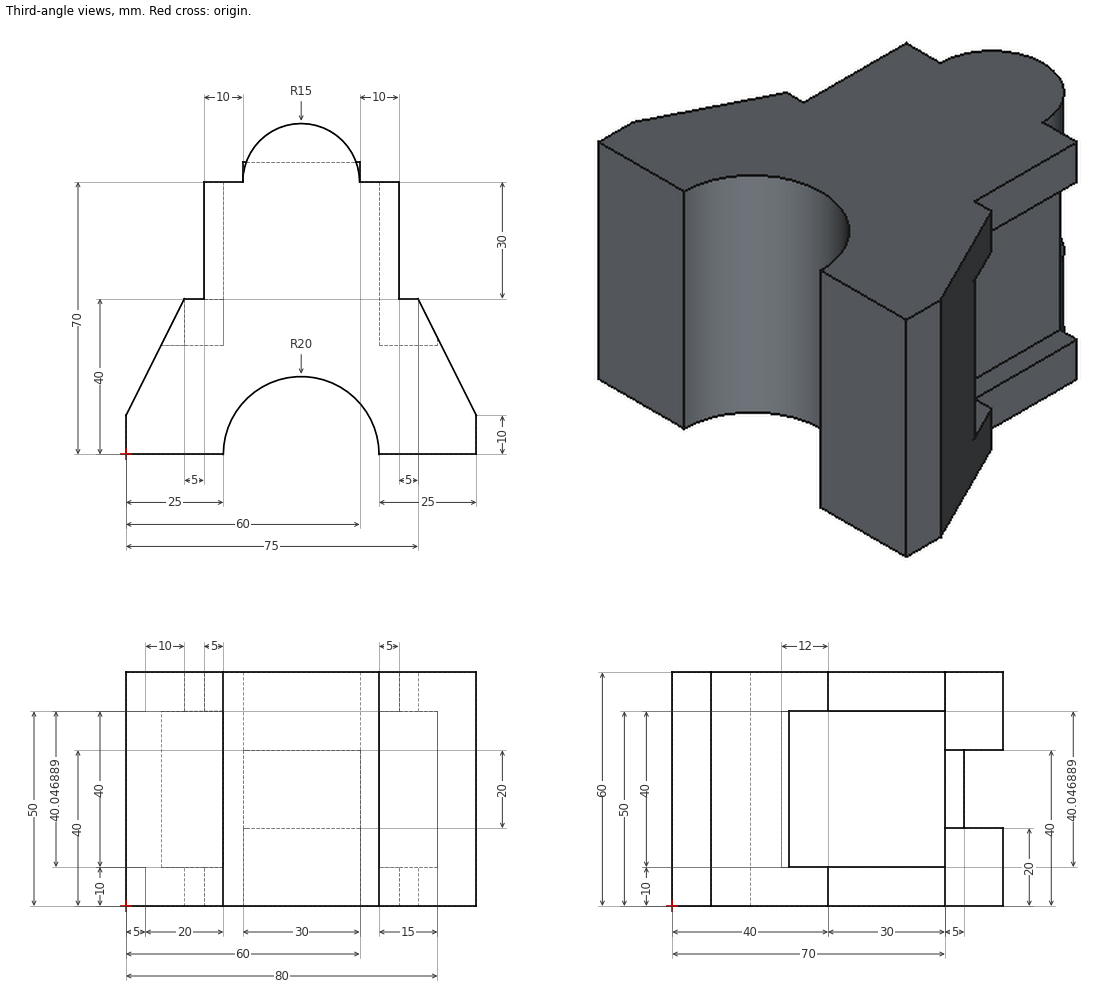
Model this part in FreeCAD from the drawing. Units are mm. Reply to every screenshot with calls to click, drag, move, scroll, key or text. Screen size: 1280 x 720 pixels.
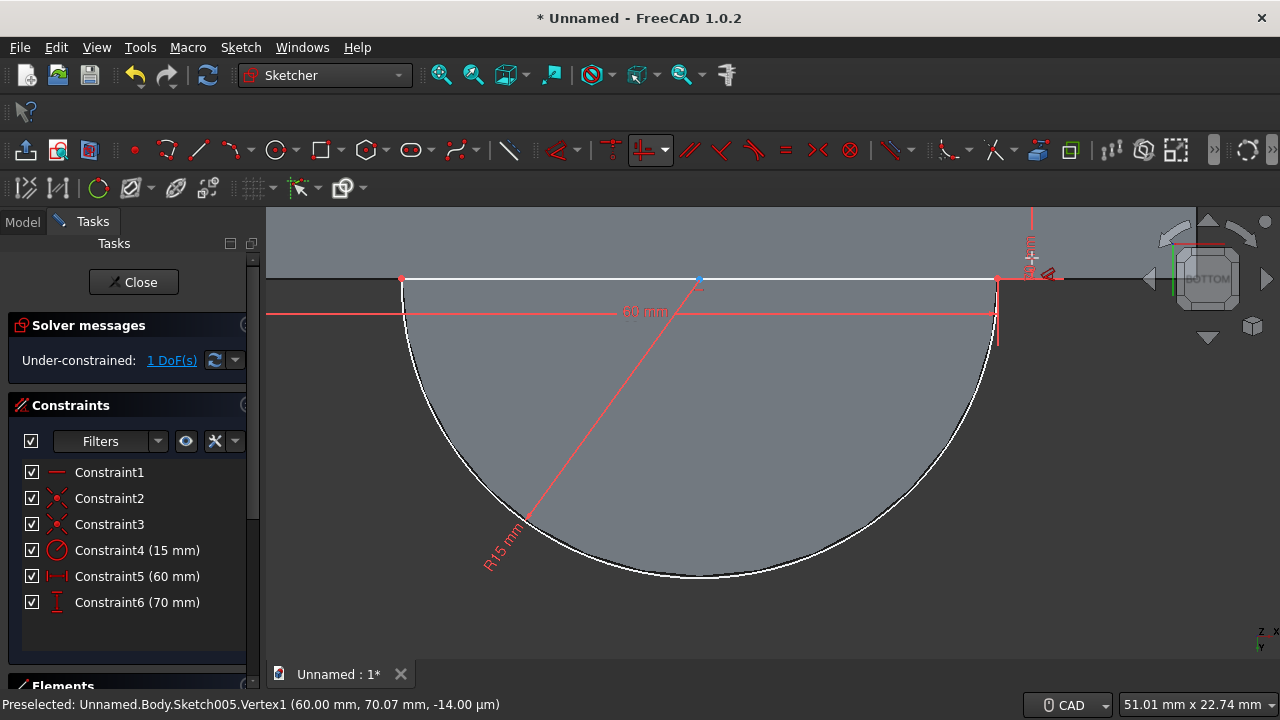
click(700, 280)
click(734, 257)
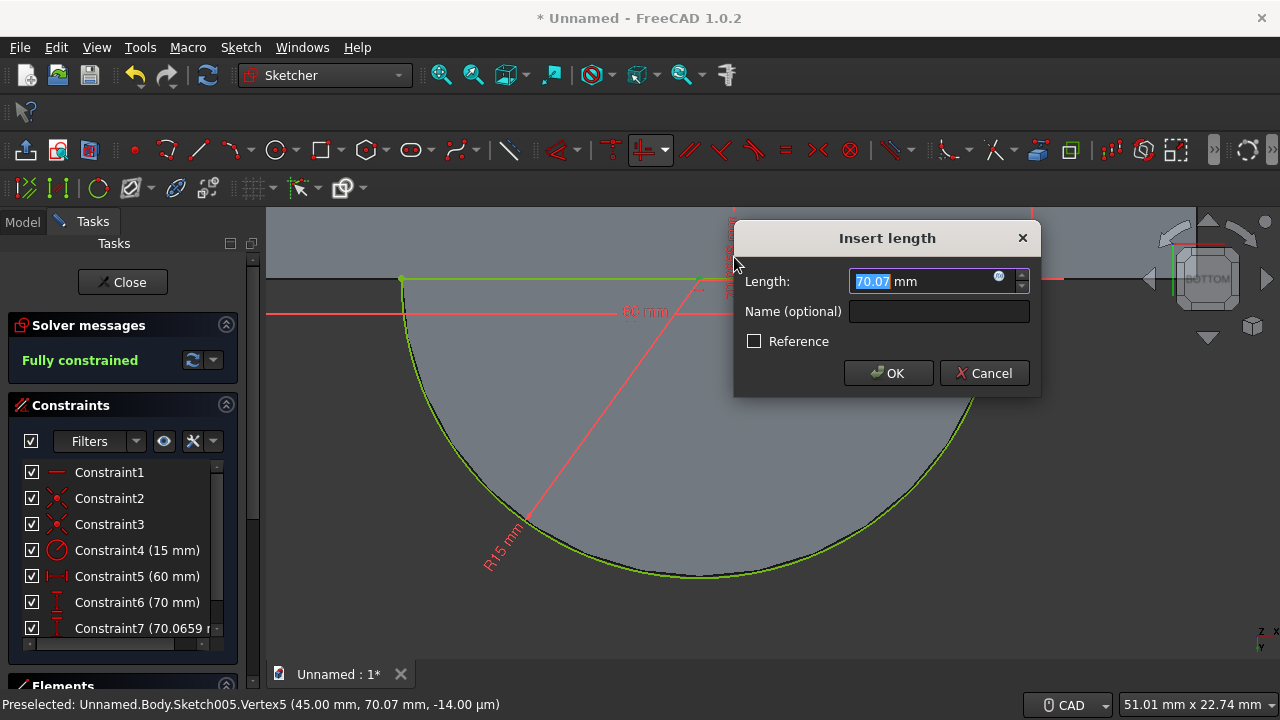
text(70)
key(Return)
key(Escape)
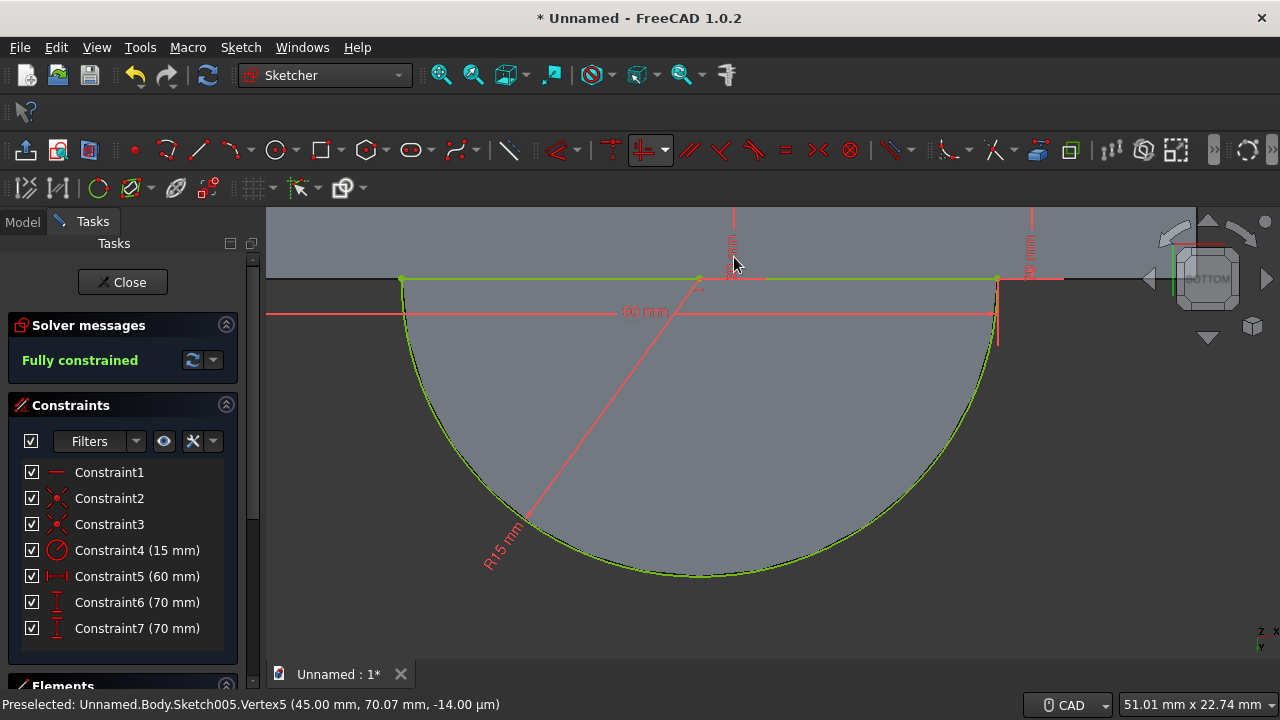
click(123, 282)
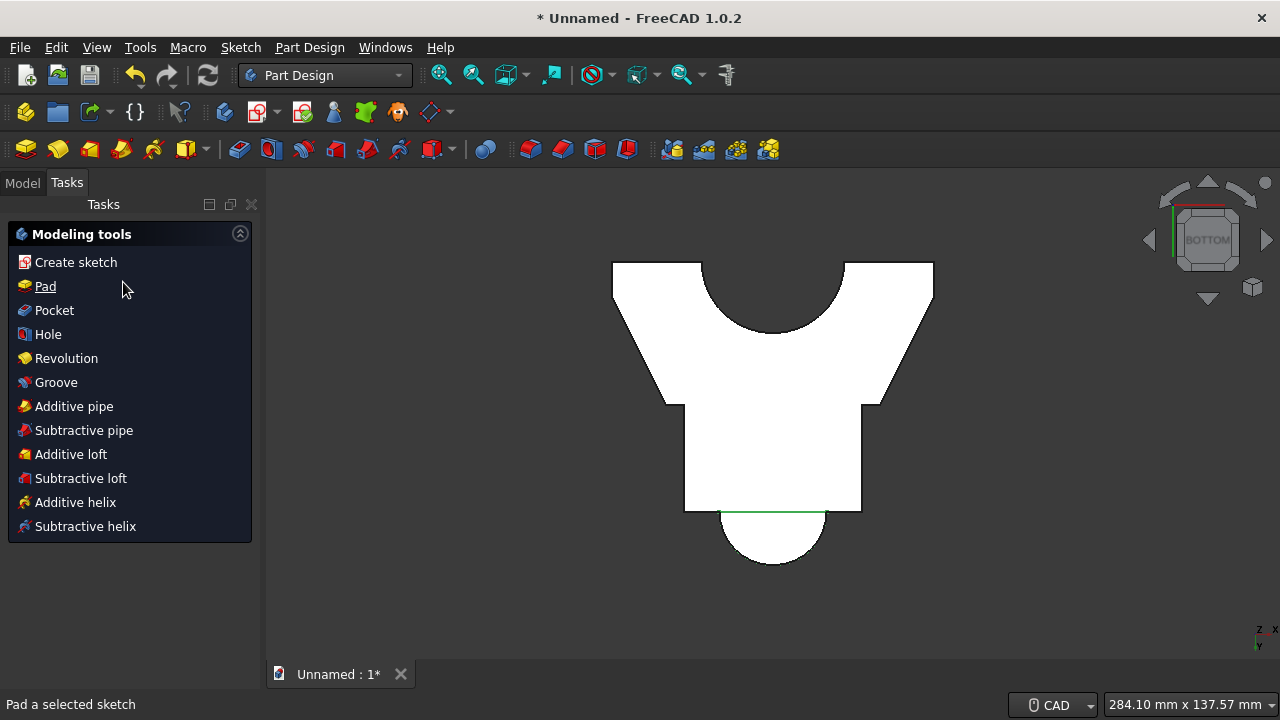
click(240, 150)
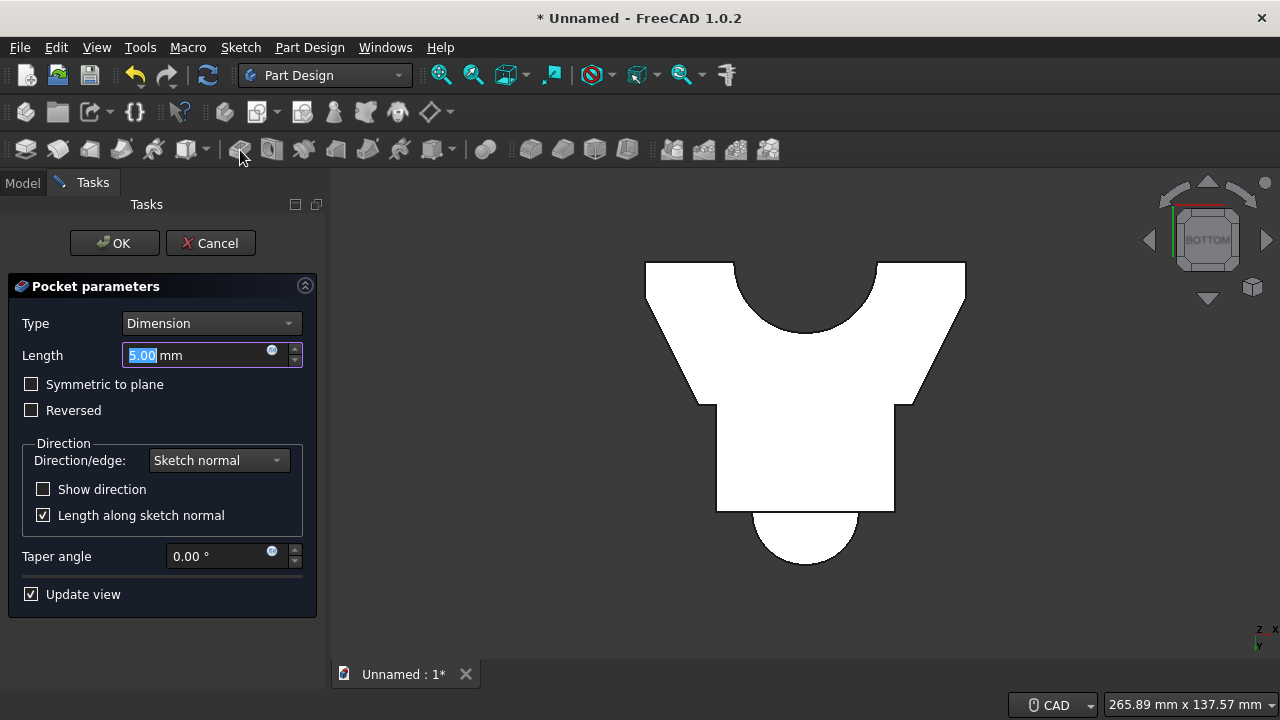
text(40)
key(Tab)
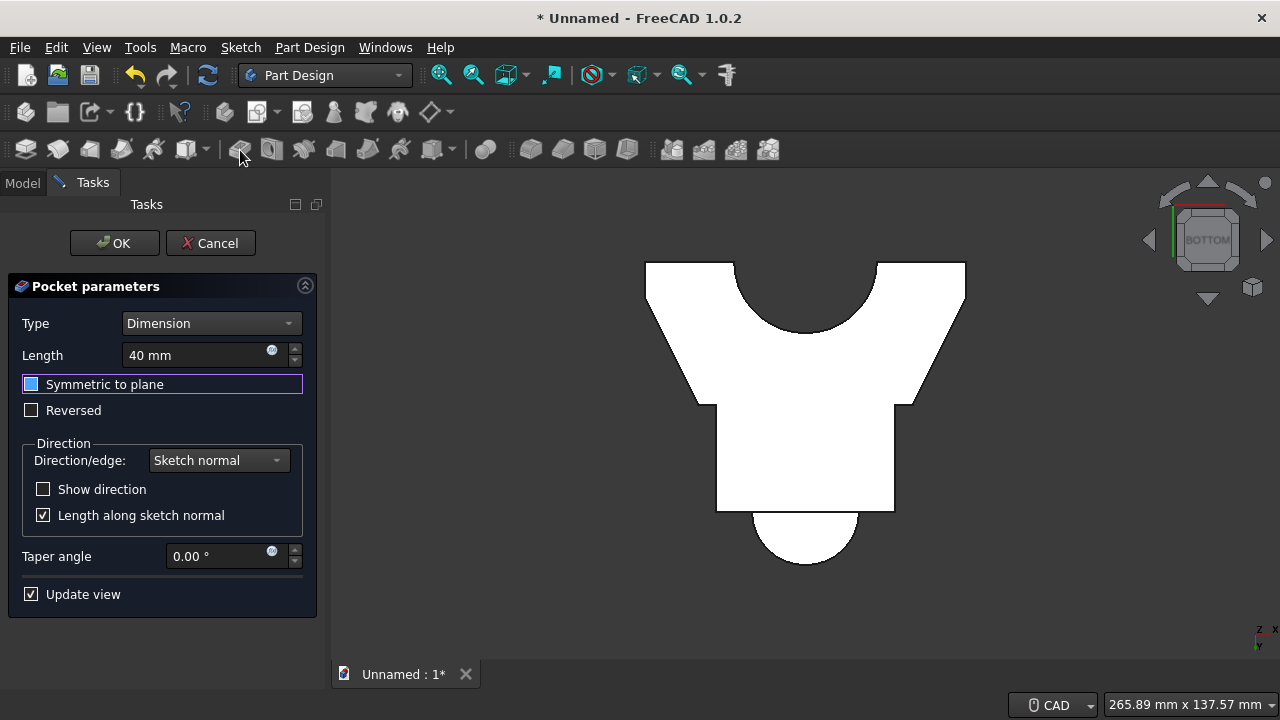
click(115, 243)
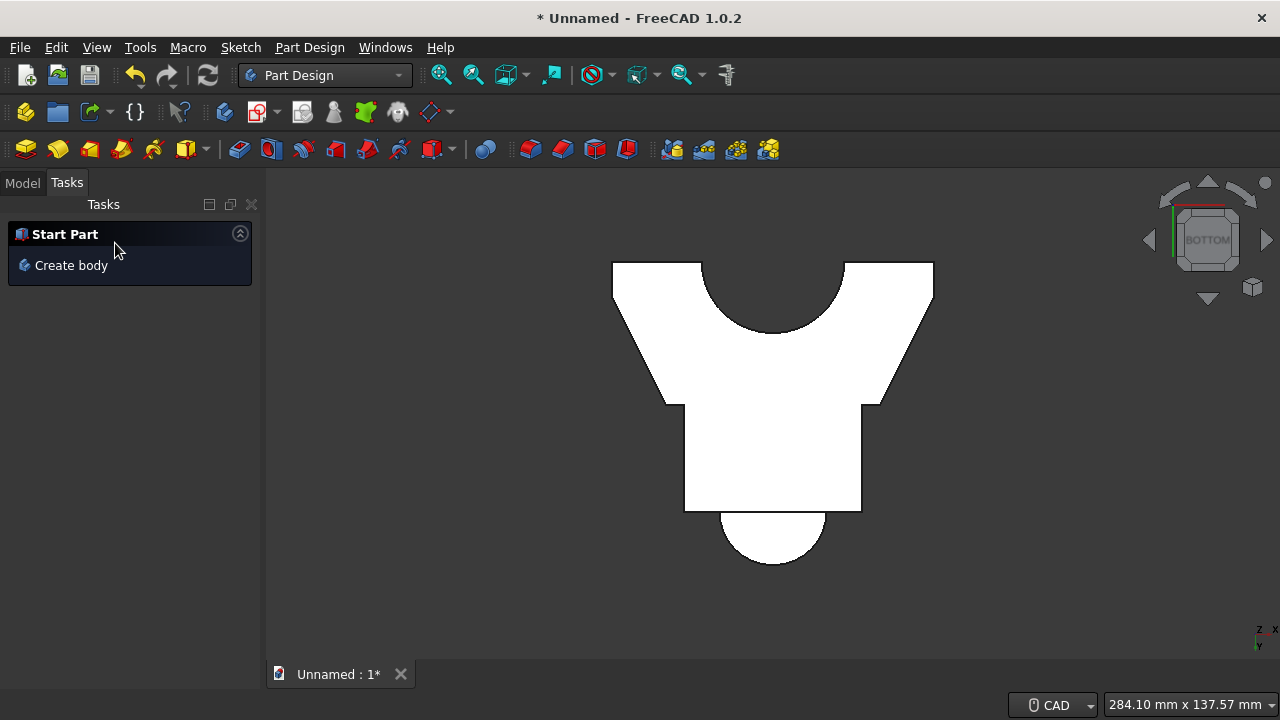
key(4)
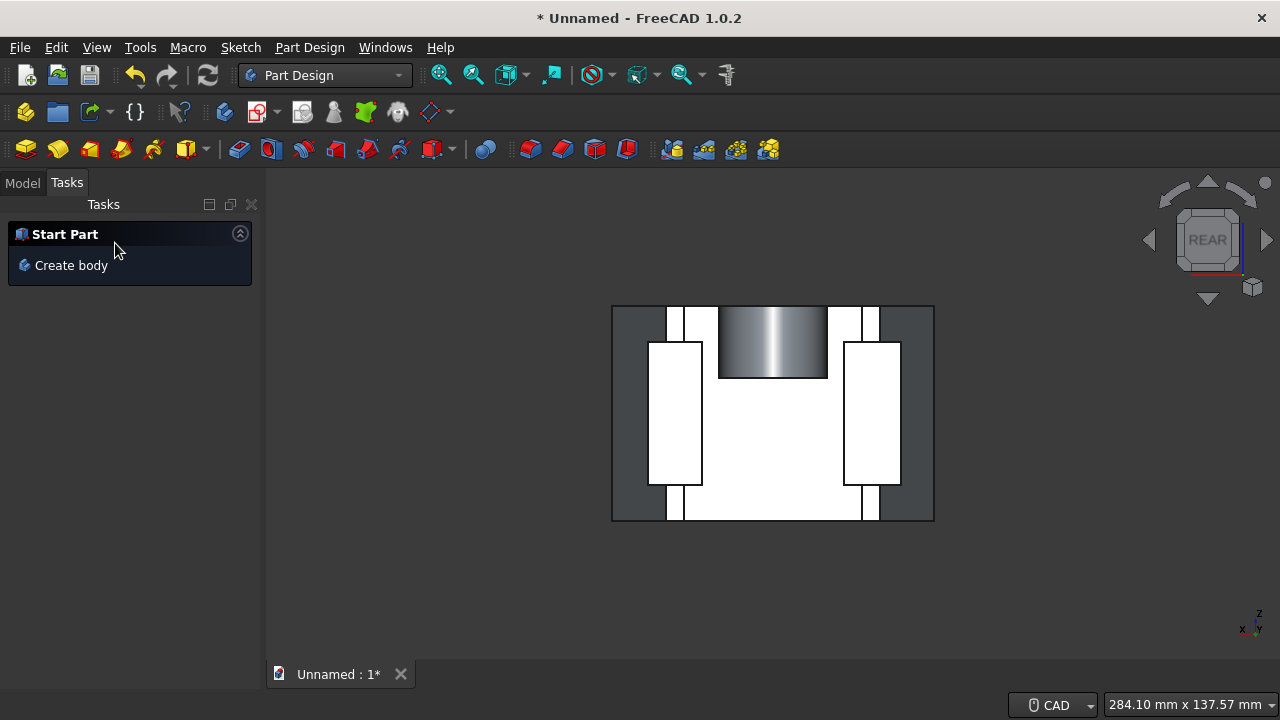
click(442, 76)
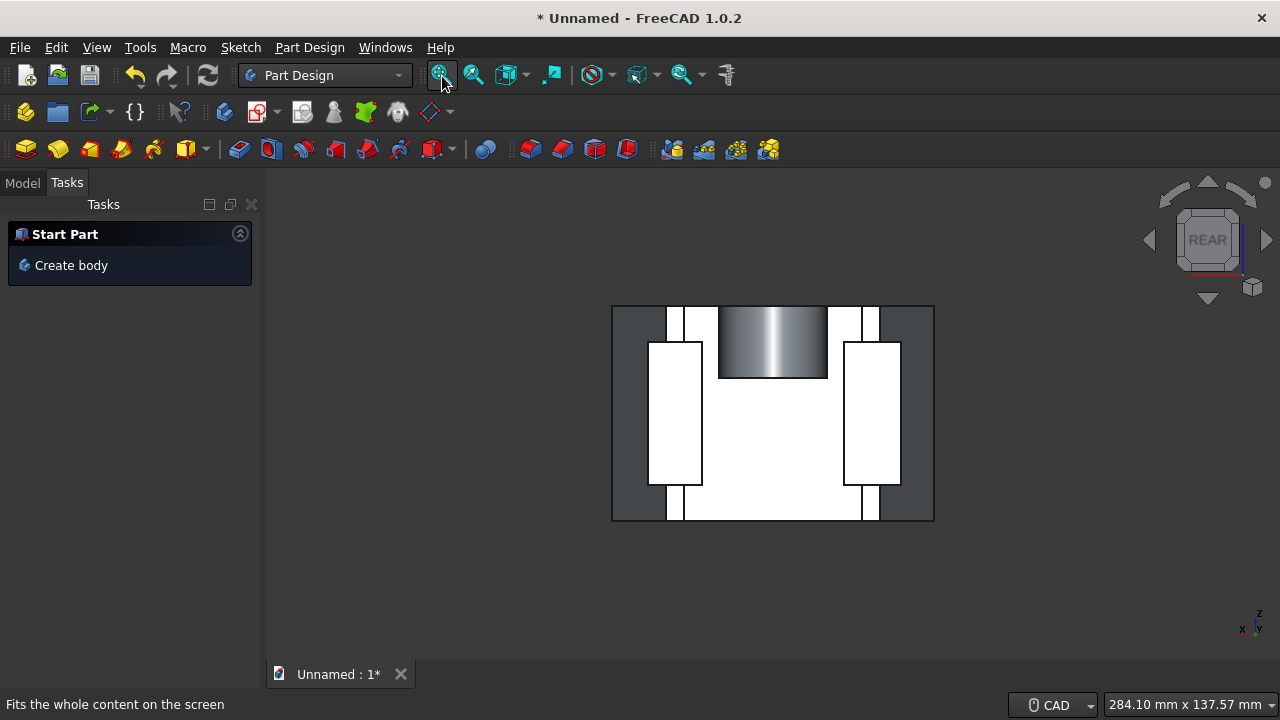
click(773, 443)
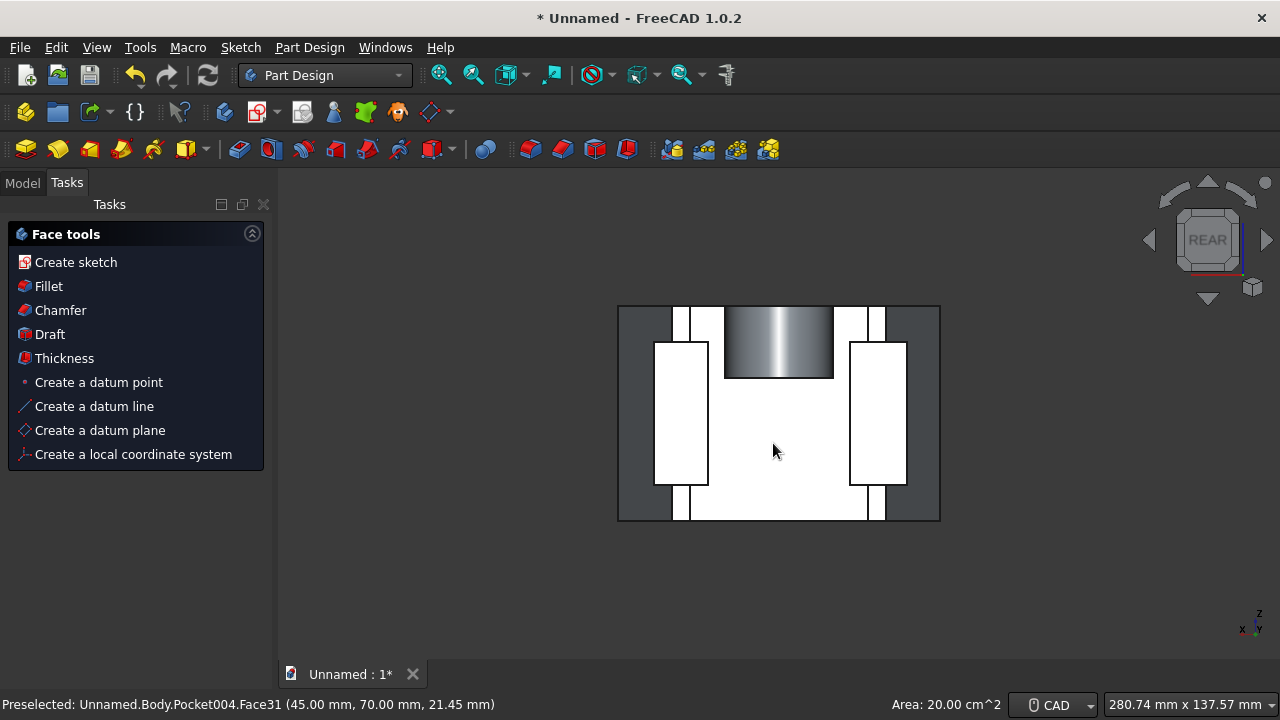
click(258, 112)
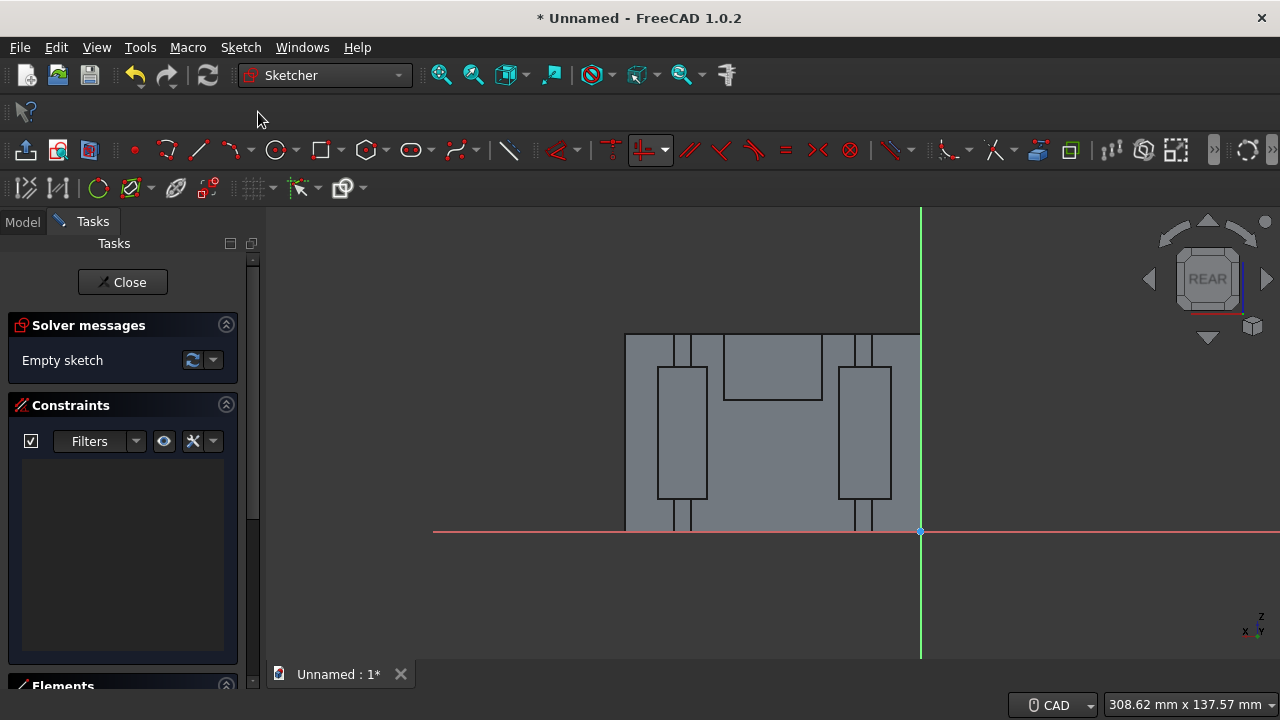
click(90, 150)